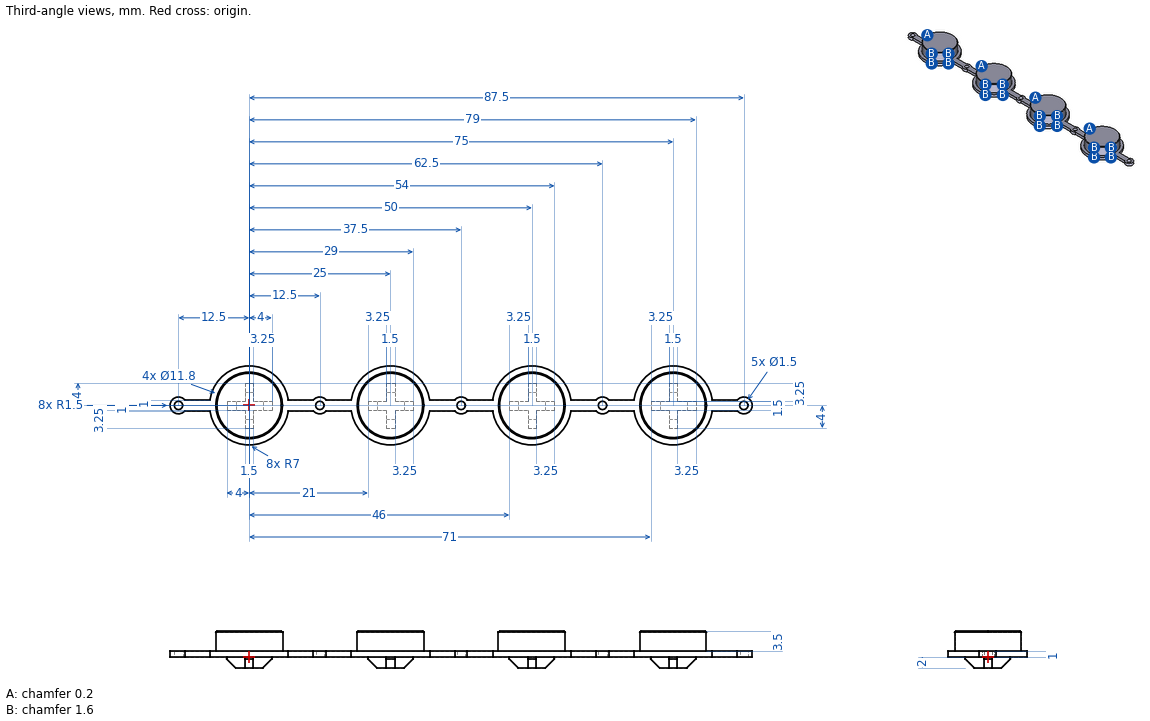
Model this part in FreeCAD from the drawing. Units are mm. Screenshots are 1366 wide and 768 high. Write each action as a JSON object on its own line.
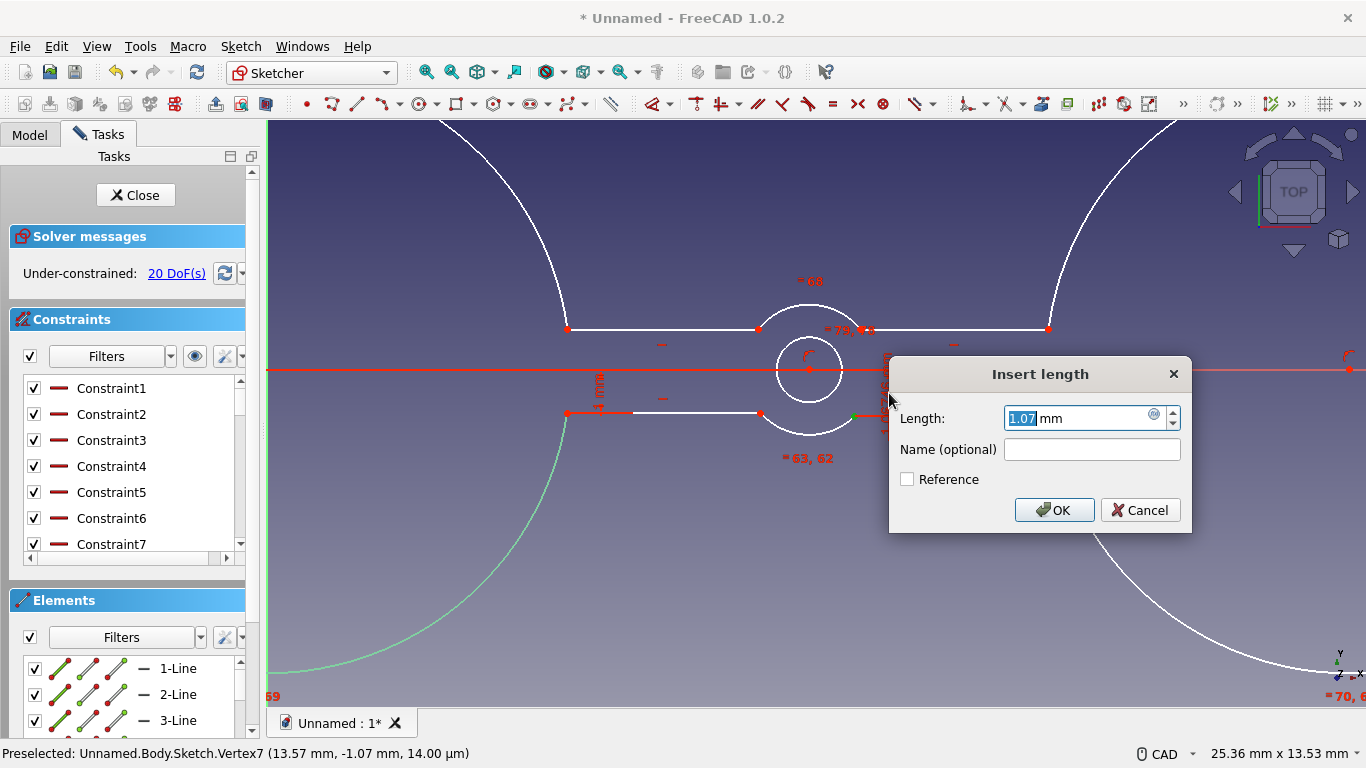
{"action": "type", "text": "1"}
{"action": "key", "text": "Return"}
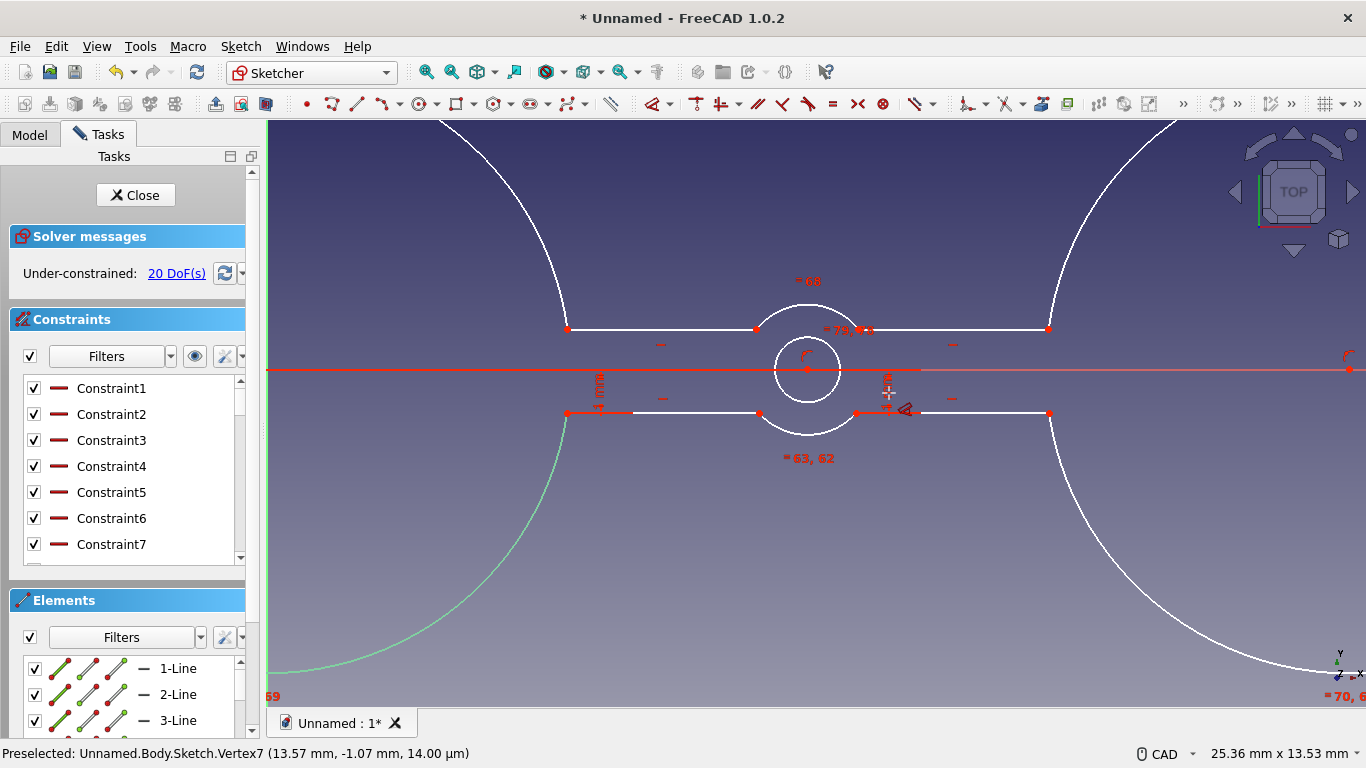
{"action": "scroll", "coordinate": [568, 420], "scroll_direction": "down", "scroll_amount": 10}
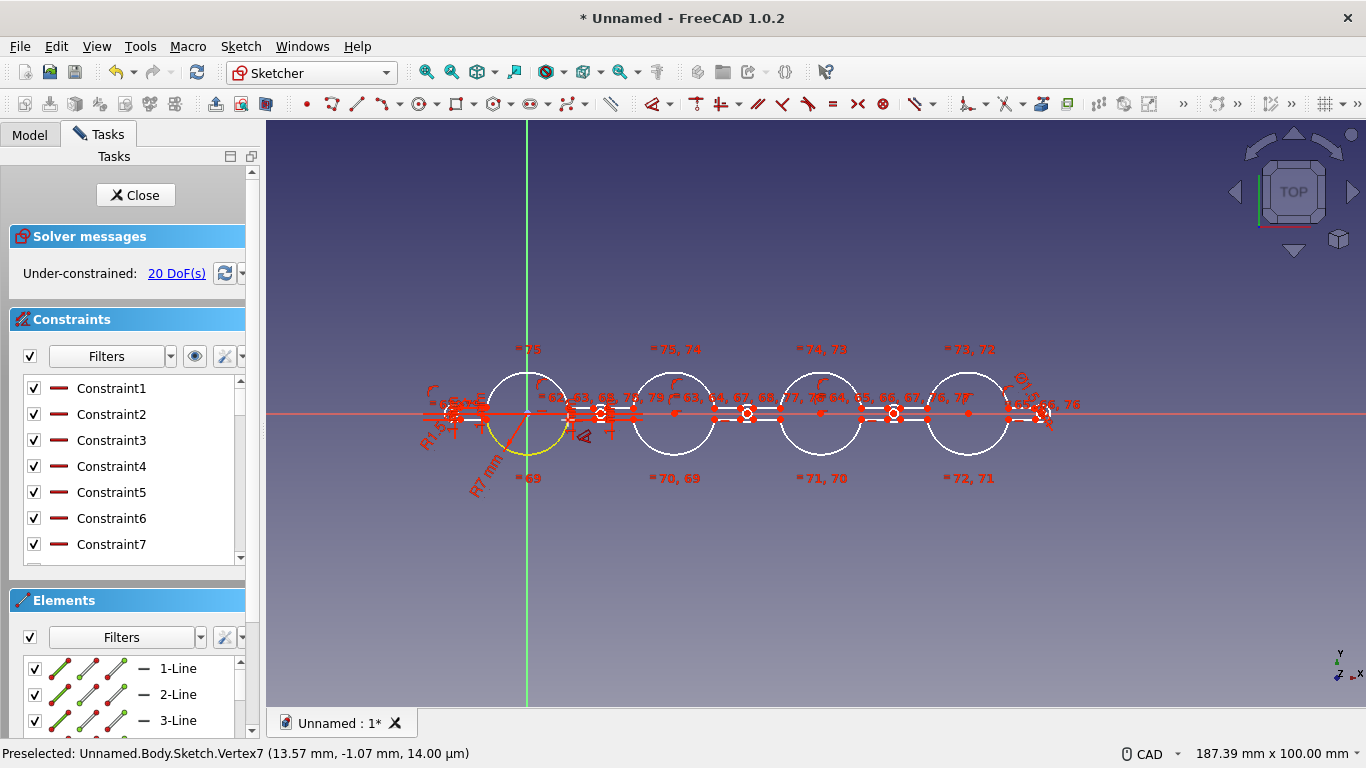
{"action": "scroll", "coordinate": [715, 420], "scroll_direction": "up", "scroll_amount": 10}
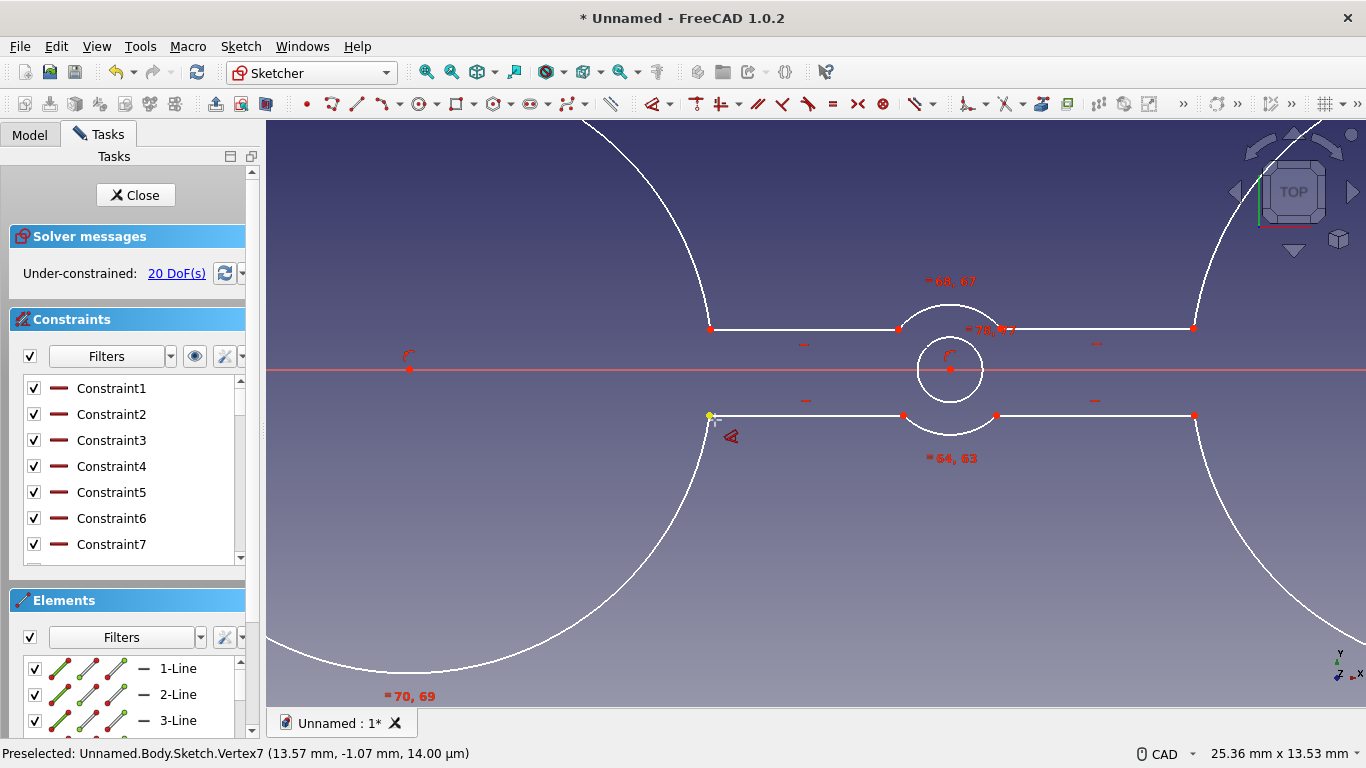
{"action": "left_click", "coordinate": [710, 416]}
{"action": "left_click", "coordinate": [744, 393]}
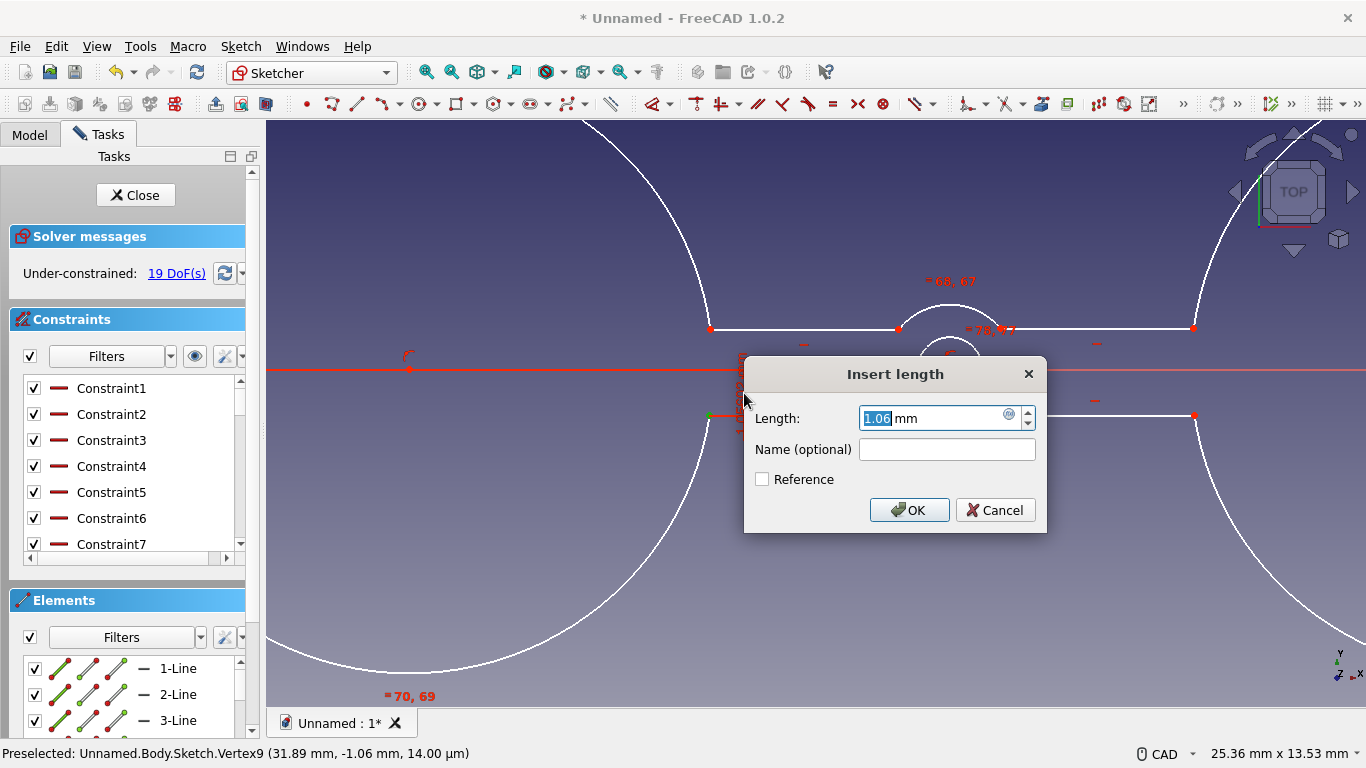
{"action": "type", "text": "1"}
{"action": "key", "text": "Return"}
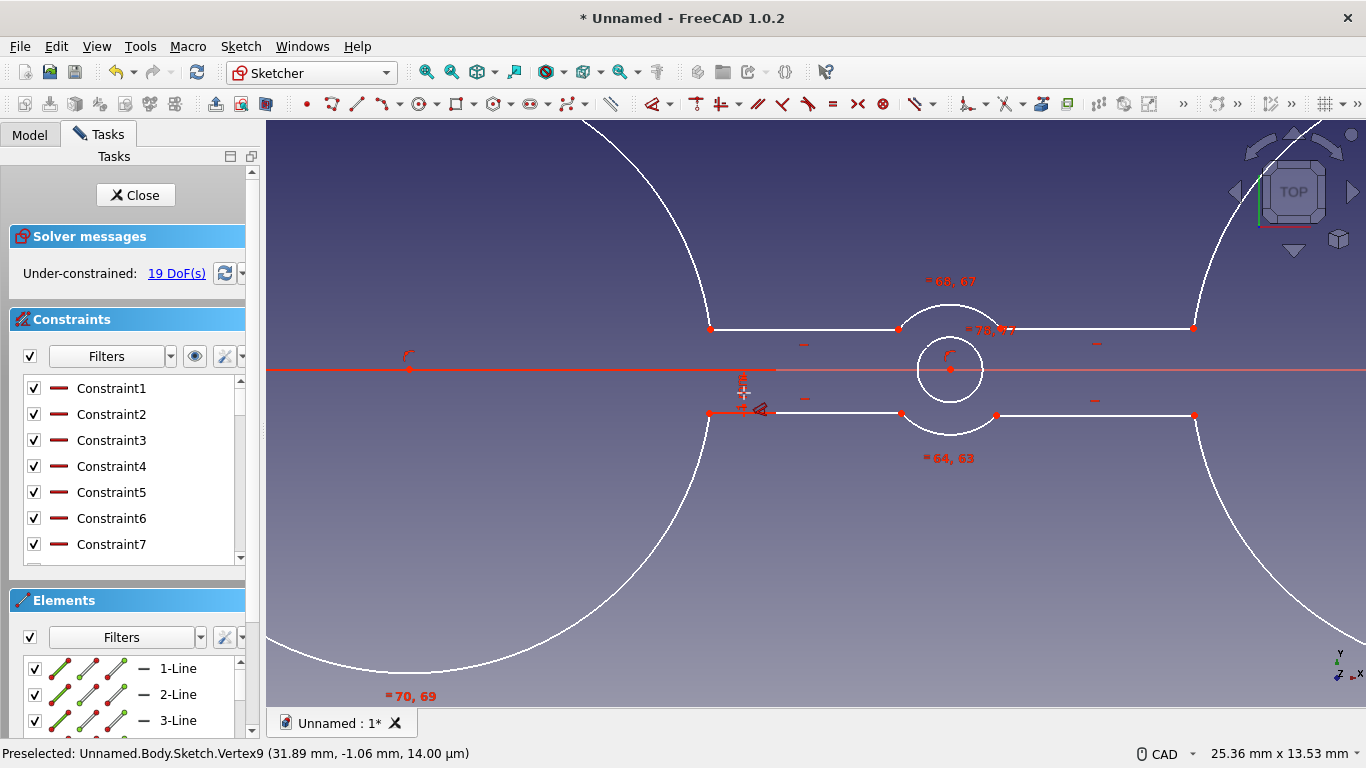
{"action": "left_click", "coordinate": [996, 416]}
{"action": "left_click", "coordinate": [1030, 393]}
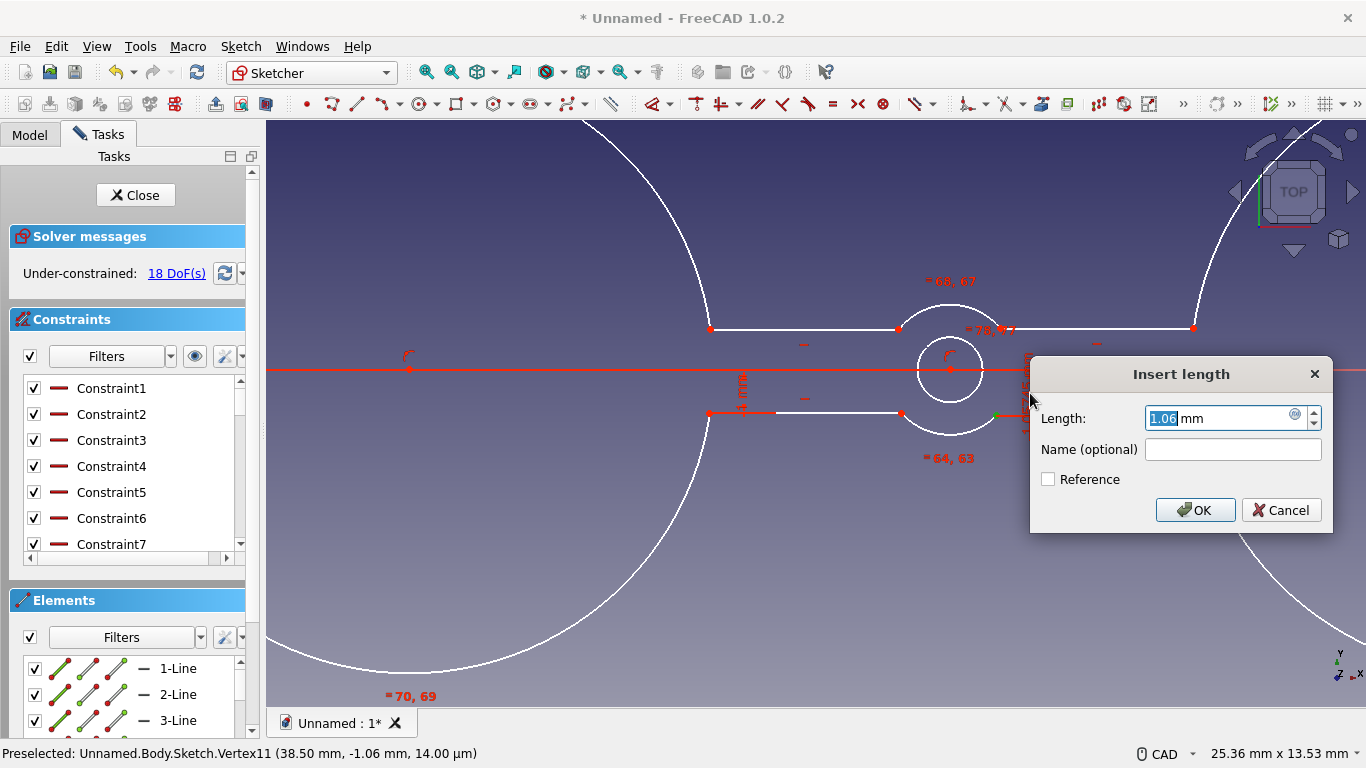
{"action": "type", "text": "1"}
{"action": "key", "text": "Return"}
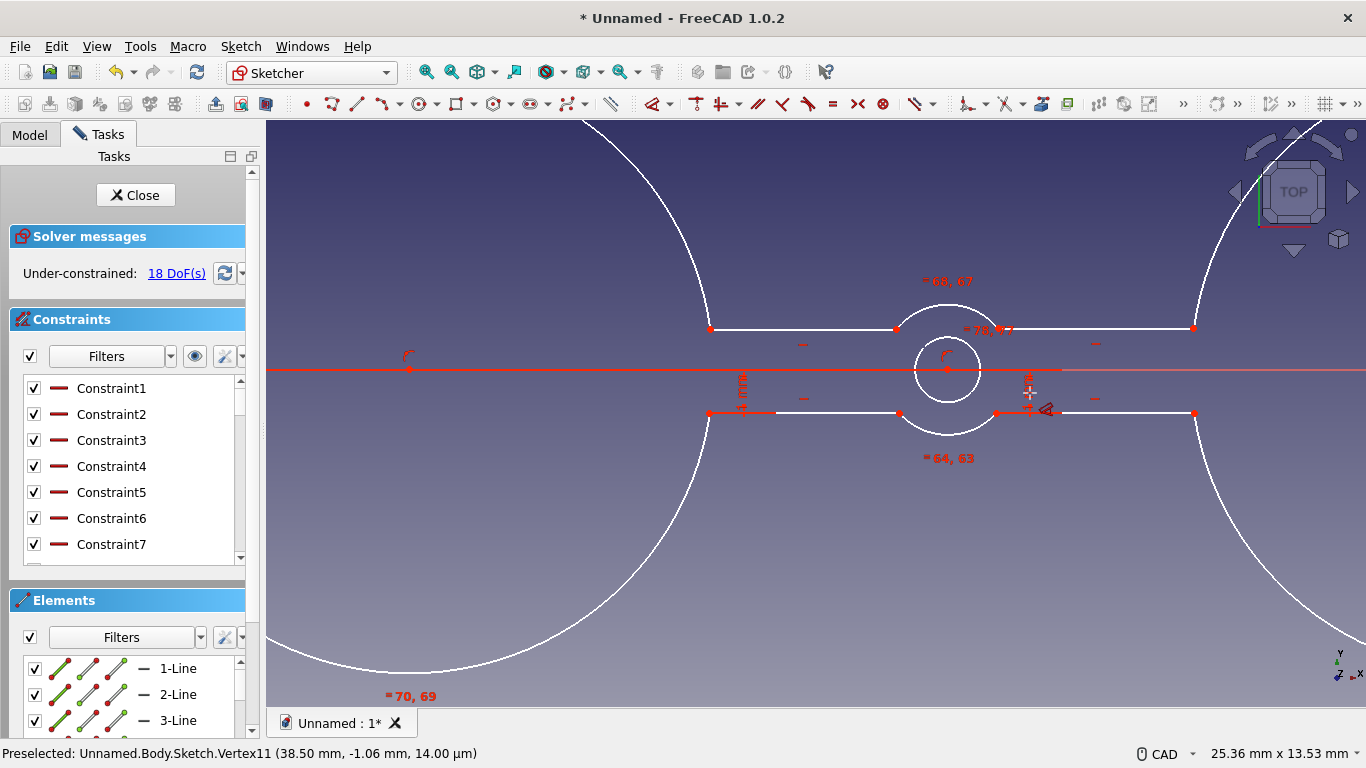
{"action": "scroll", "coordinate": [715, 420], "scroll_direction": "down", "scroll_amount": 10}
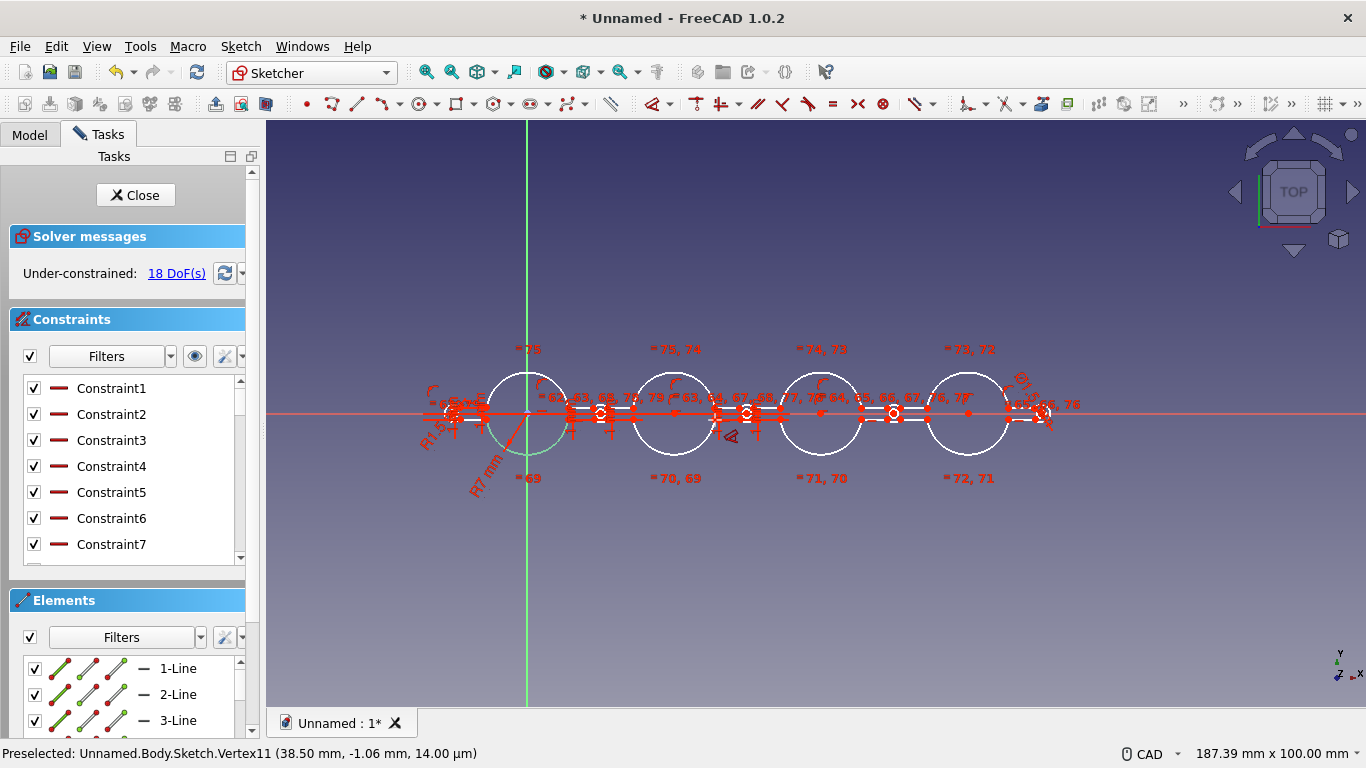
{"action": "scroll", "coordinate": [861, 420], "scroll_direction": "up", "scroll_amount": 10}